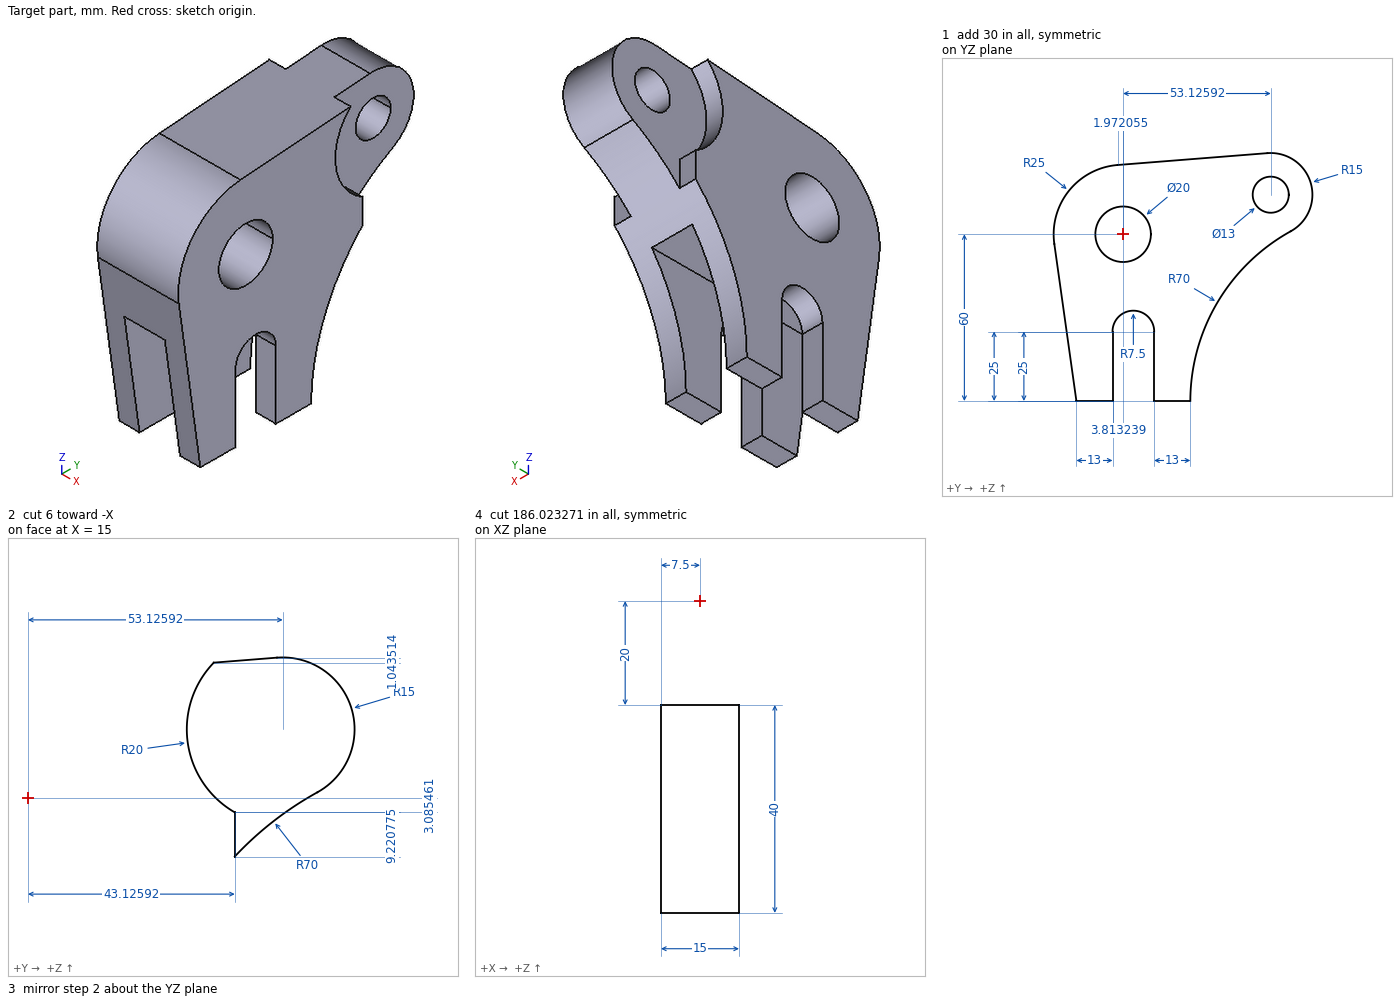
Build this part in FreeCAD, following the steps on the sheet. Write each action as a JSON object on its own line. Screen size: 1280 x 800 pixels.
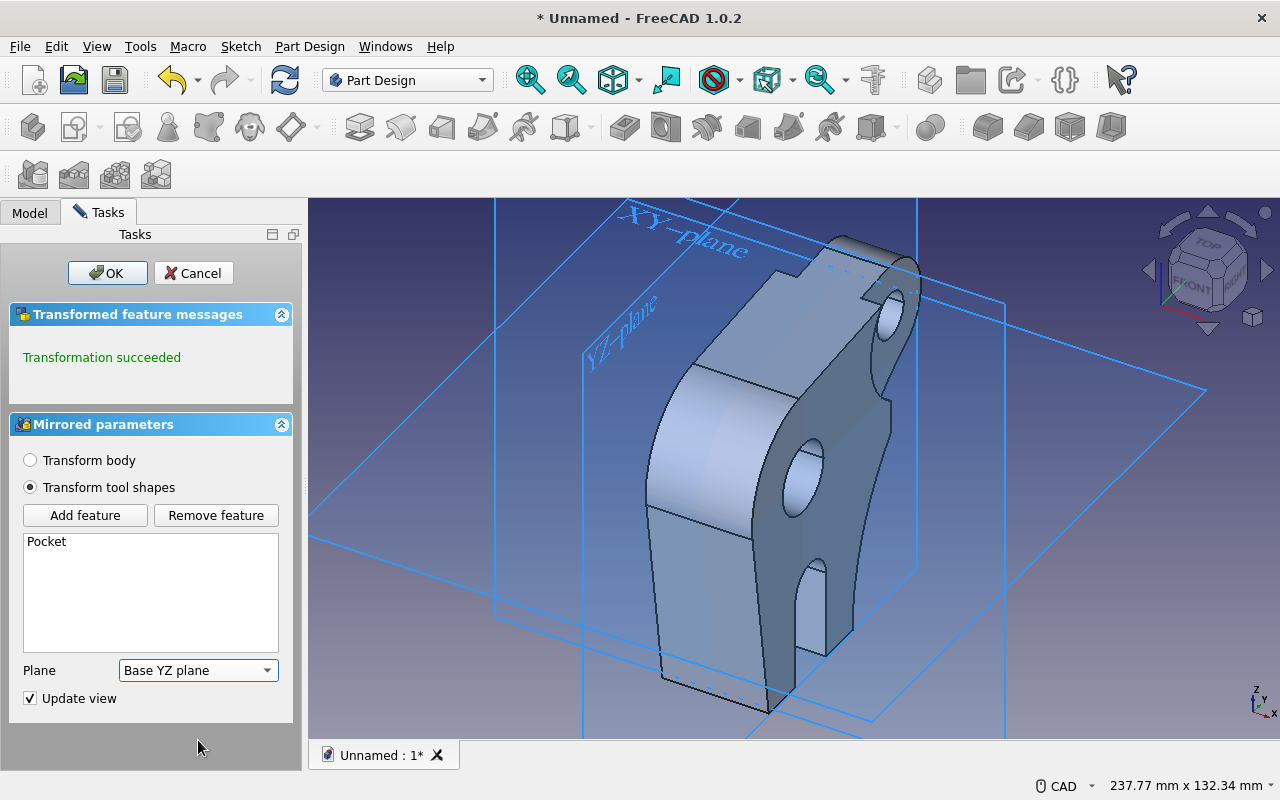
{"action": "left_click", "coordinate": [108, 273]}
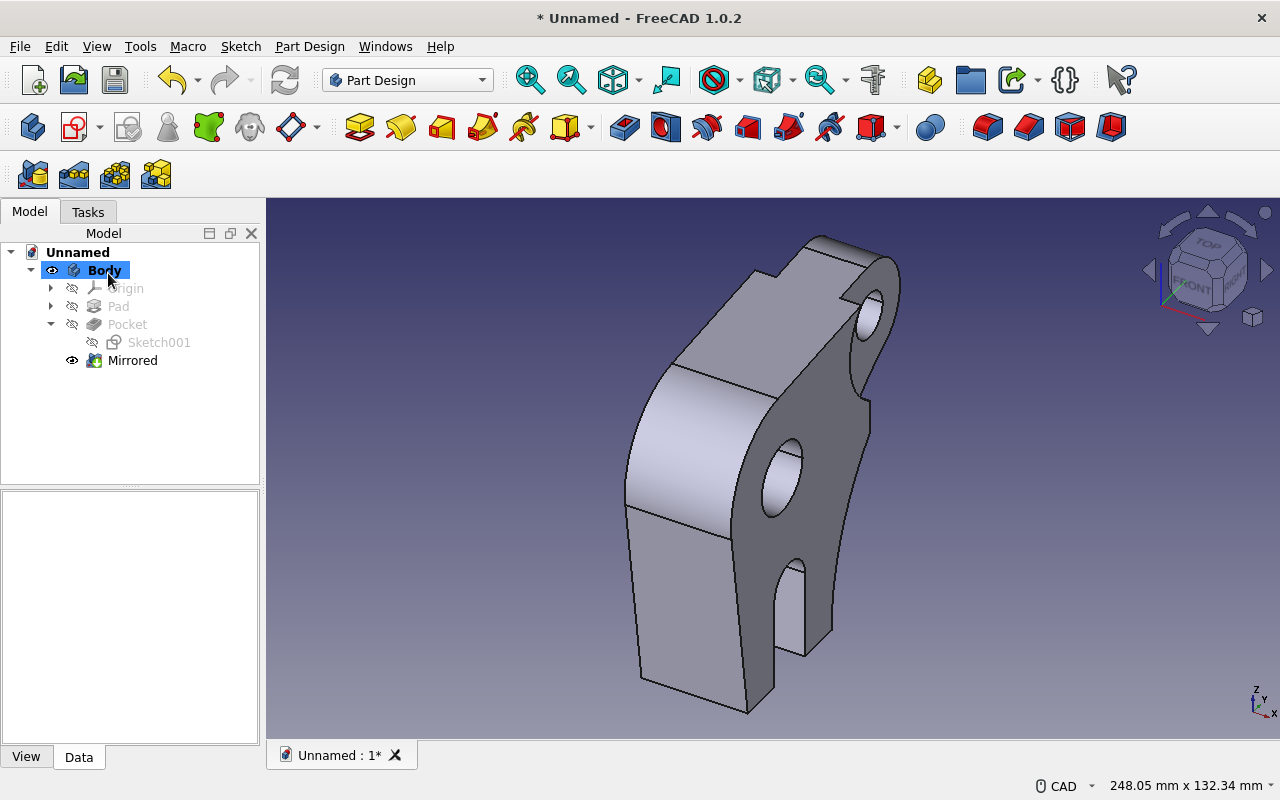
{"action": "left_click", "coordinate": [74, 128]}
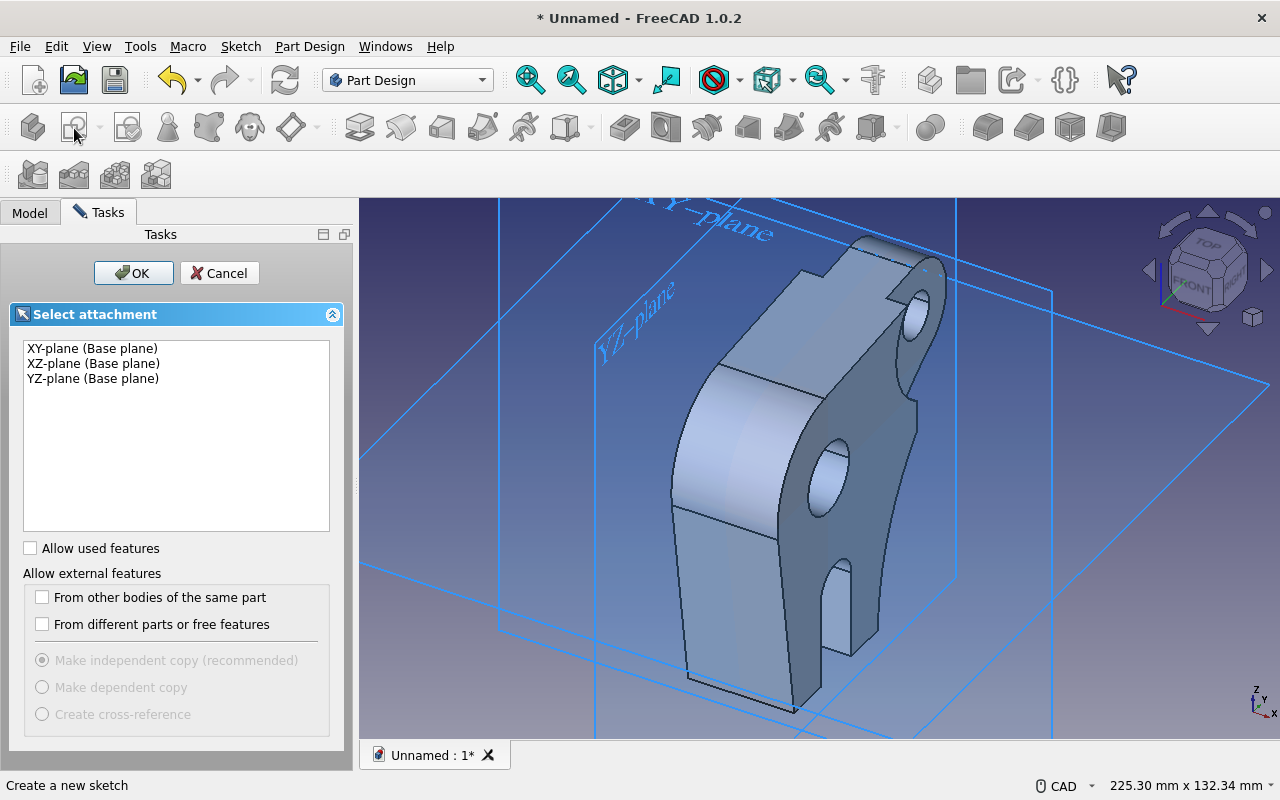
{"action": "left_click", "coordinate": [84, 364]}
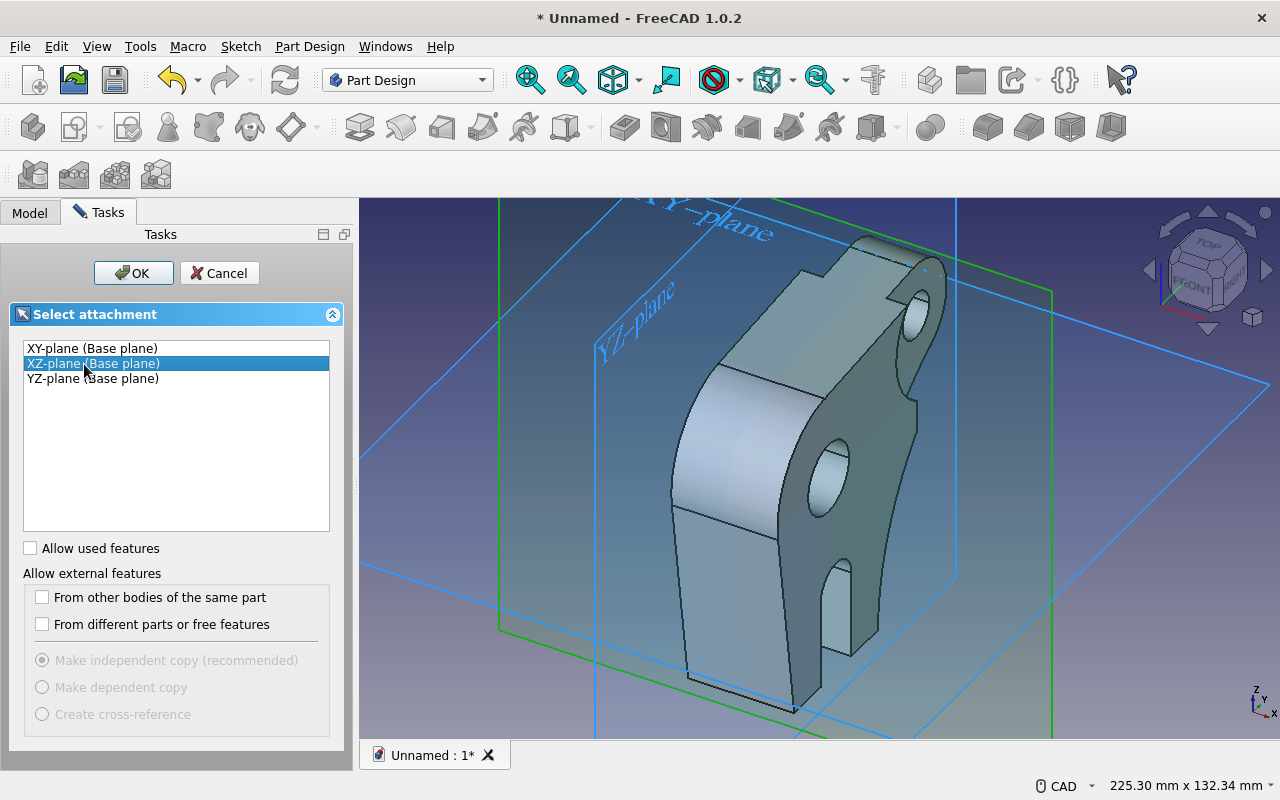
{"action": "left_click", "coordinate": [134, 273]}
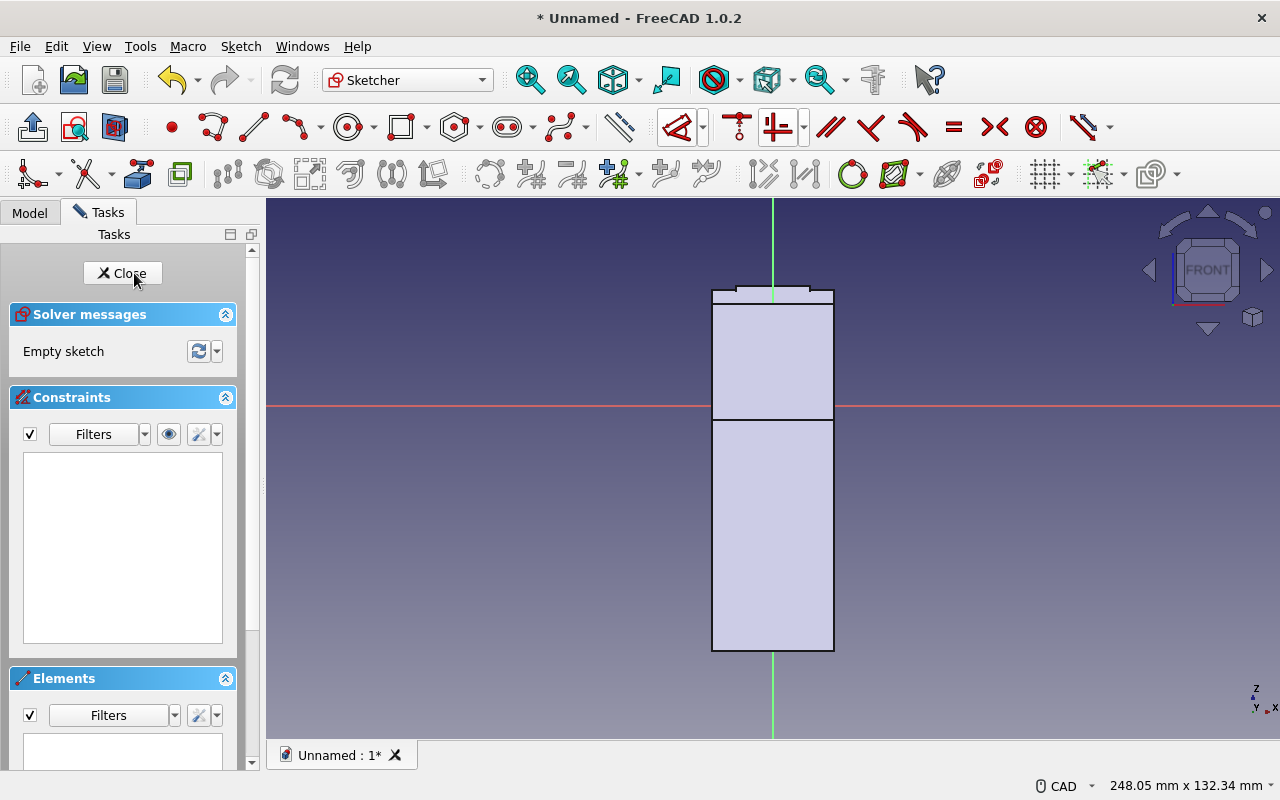
{"action": "left_click", "coordinate": [115, 128]}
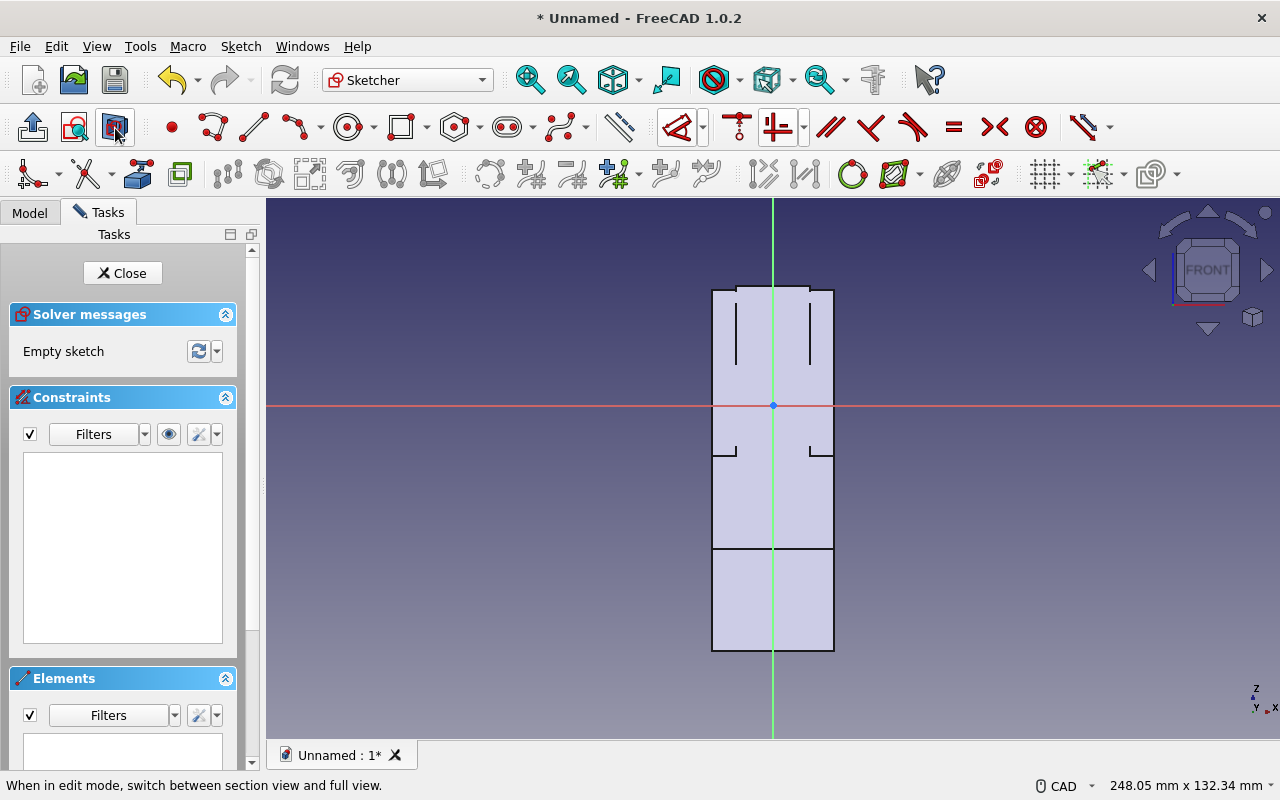
{"action": "scroll", "coordinate": [912, 649], "scroll_direction": "up", "scroll_amount": 2}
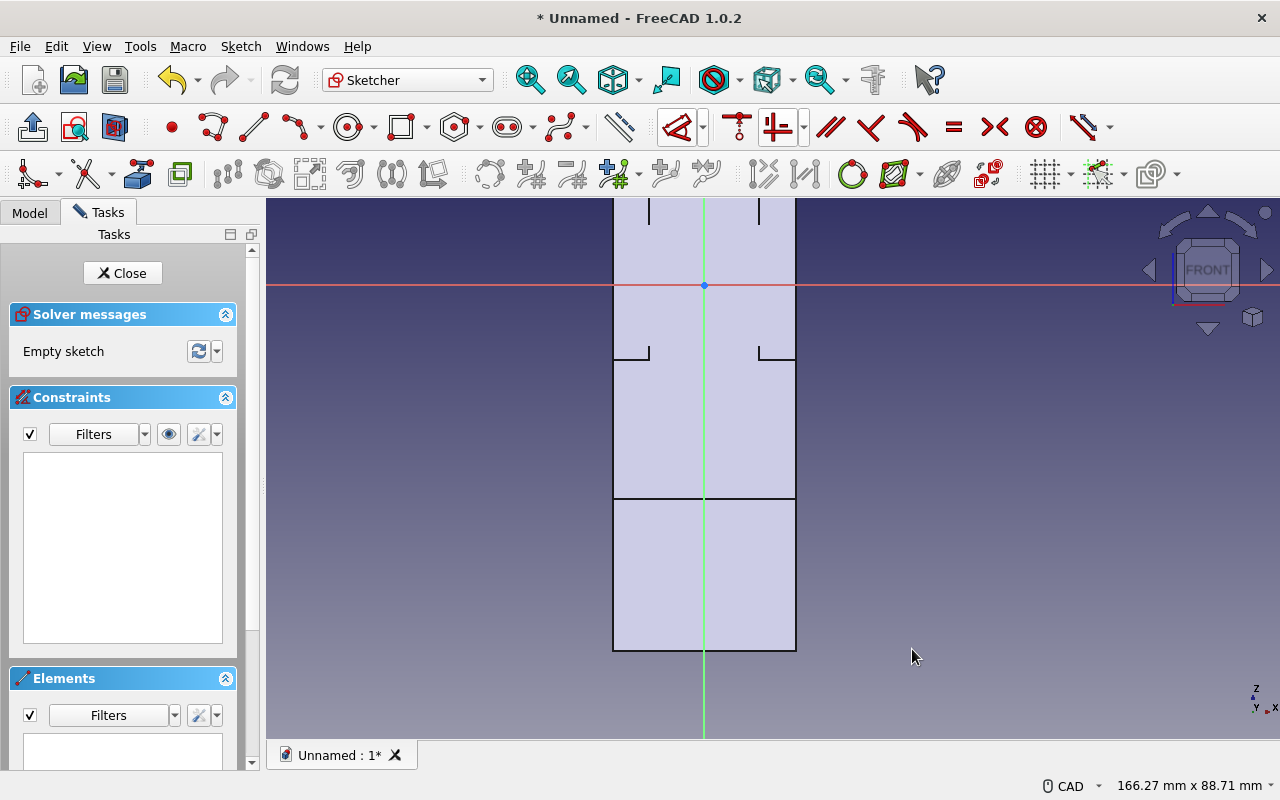
{"action": "left_click", "coordinate": [400, 128]}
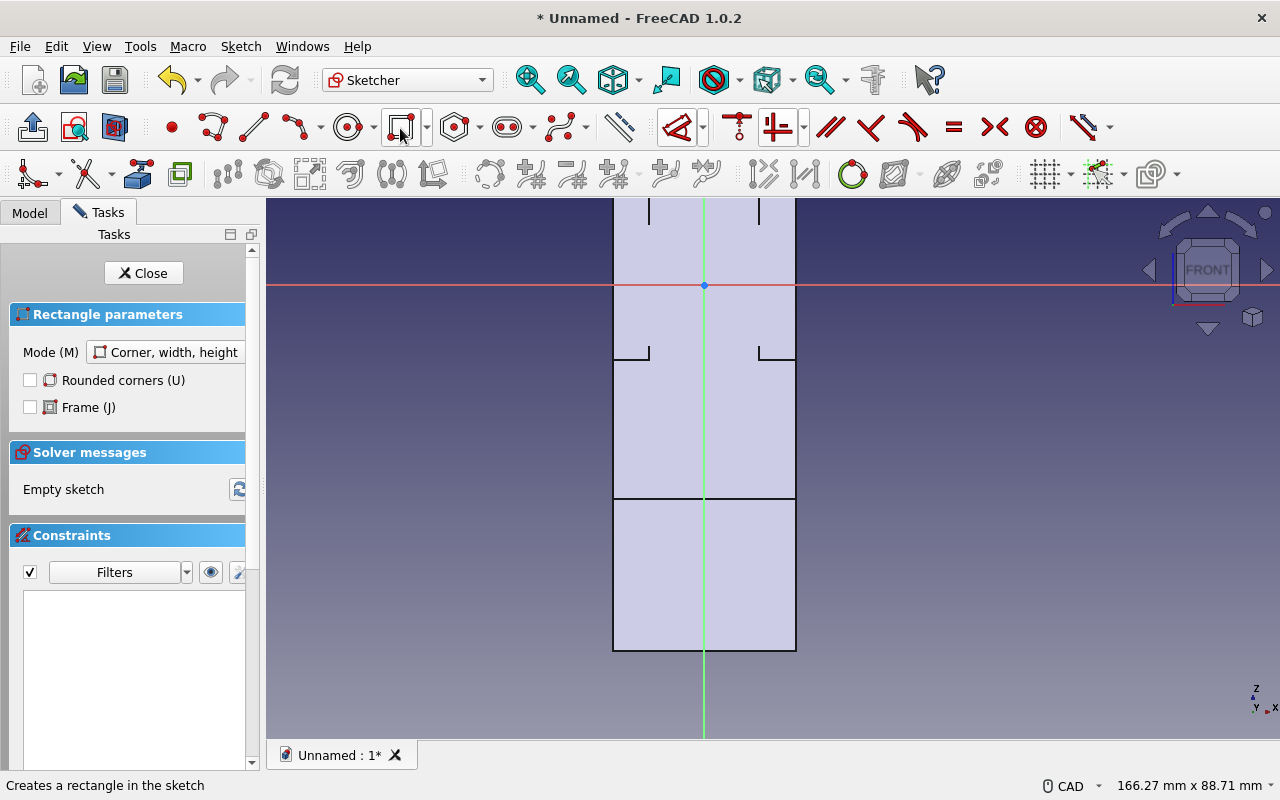
{"action": "left_click", "coordinate": [659, 407]}
{"action": "mouse_move", "coordinate": [750, 651]}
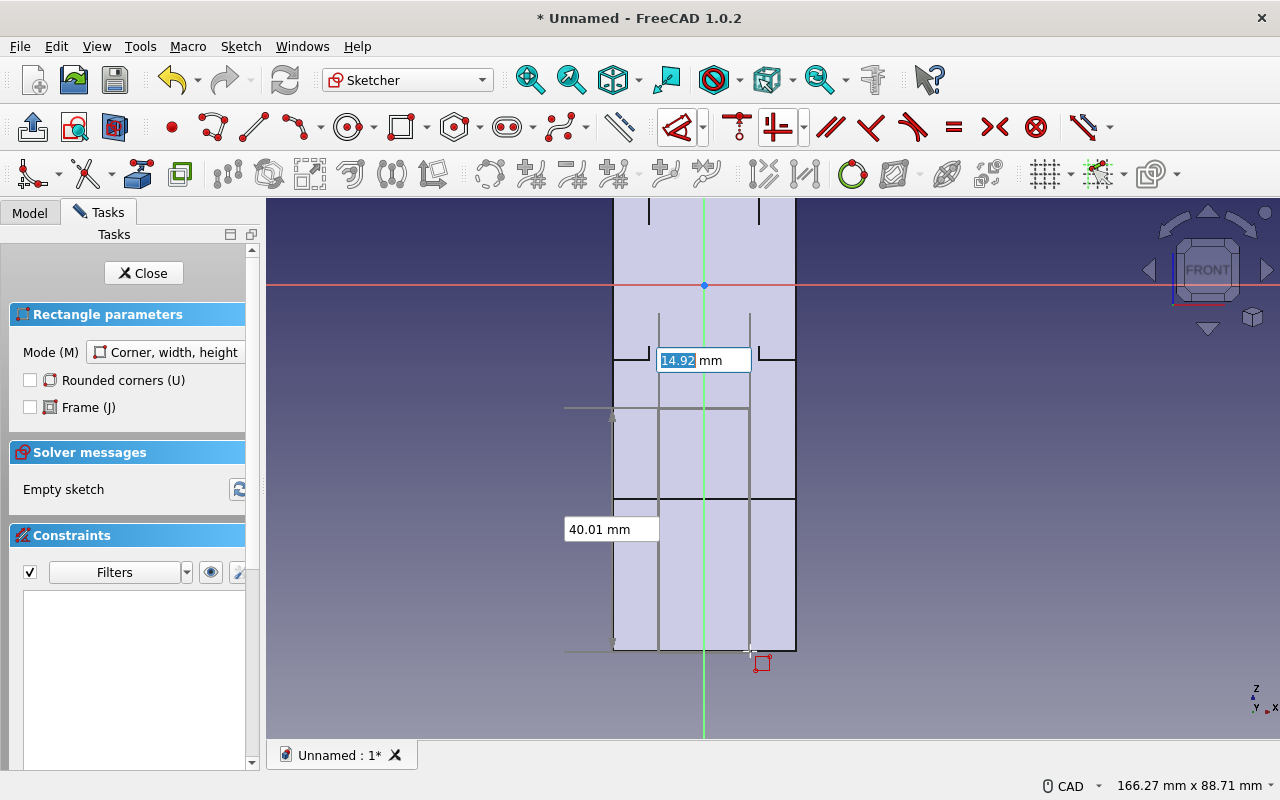
{"action": "type", "text": "15"}
{"action": "key", "text": "Tab"}
{"action": "type", "text": "40"}
{"action": "key", "text": "Return"}
{"action": "key", "text": "Escape"}